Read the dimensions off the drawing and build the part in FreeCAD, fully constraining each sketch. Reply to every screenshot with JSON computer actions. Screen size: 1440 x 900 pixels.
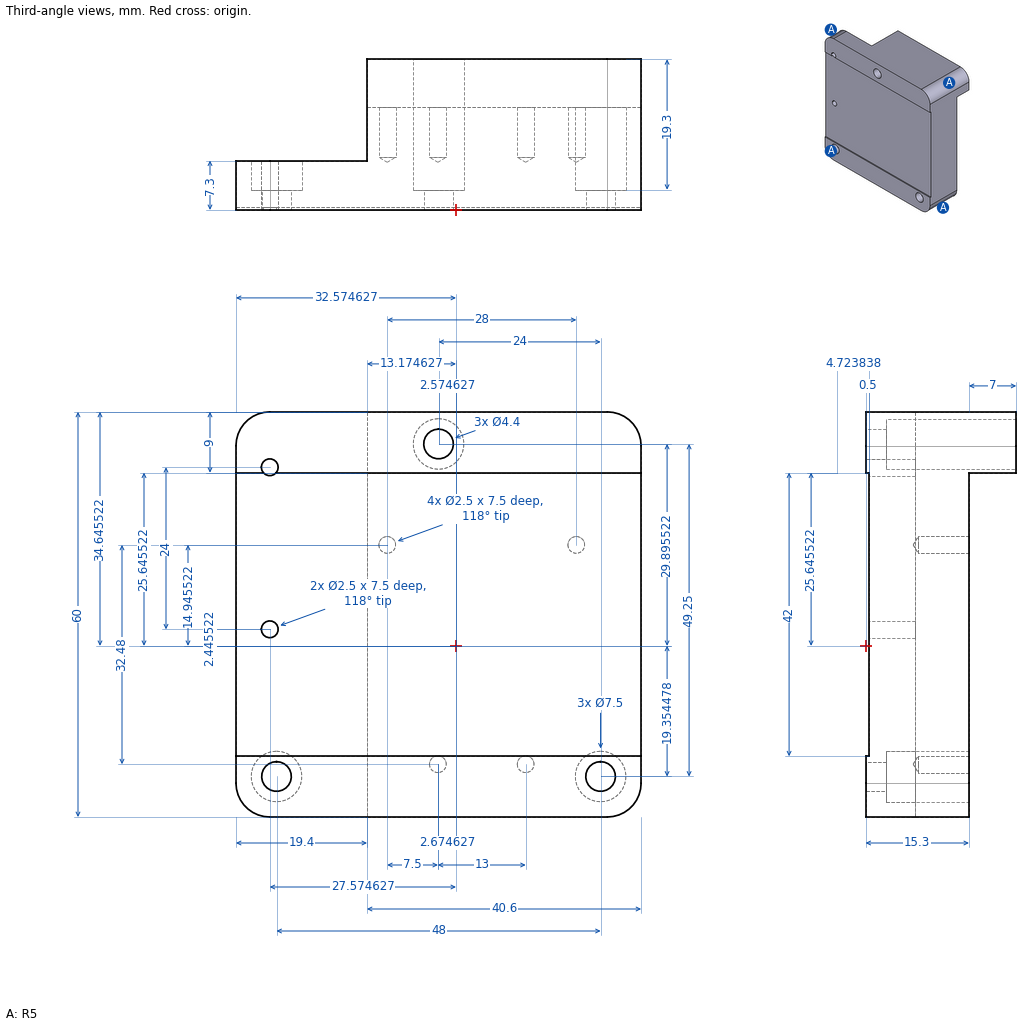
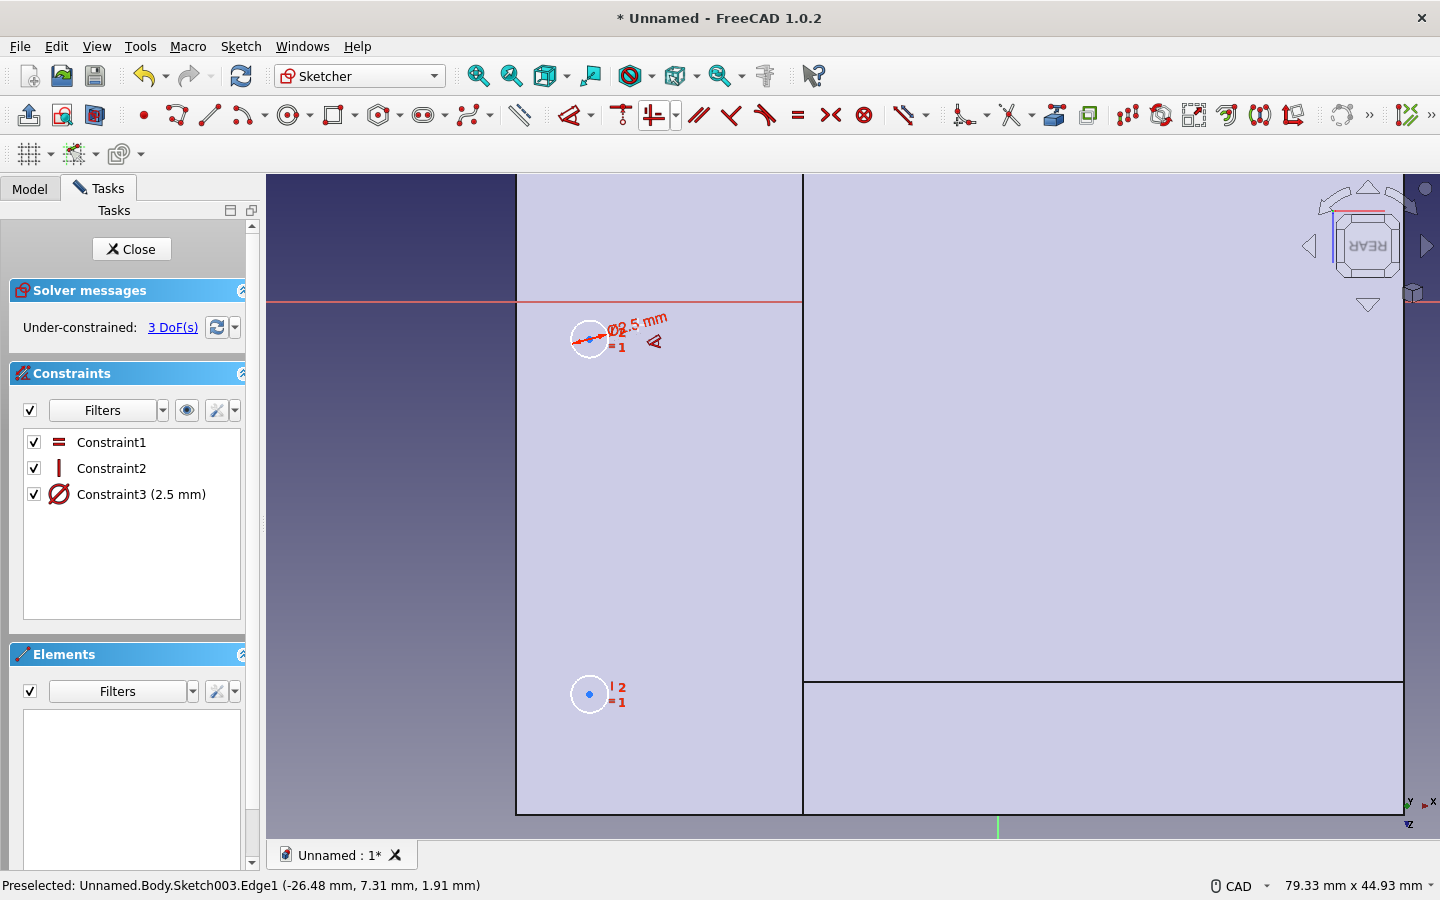
{"action": "left_click", "coordinate": [590, 339]}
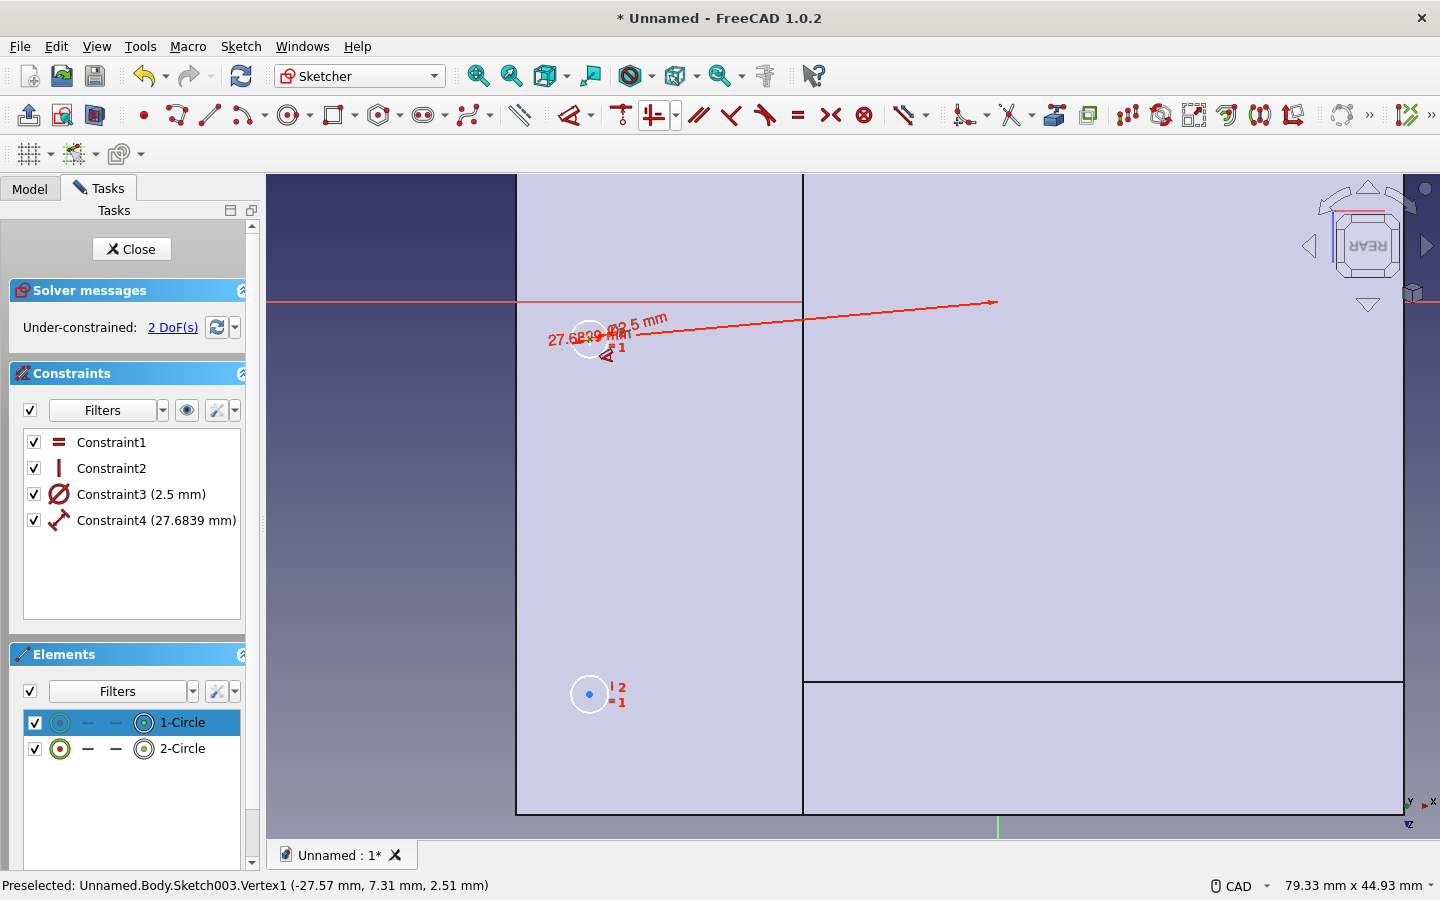
{"action": "left_click", "coordinate": [590, 694]}
{"action": "left_click", "coordinate": [556, 517]}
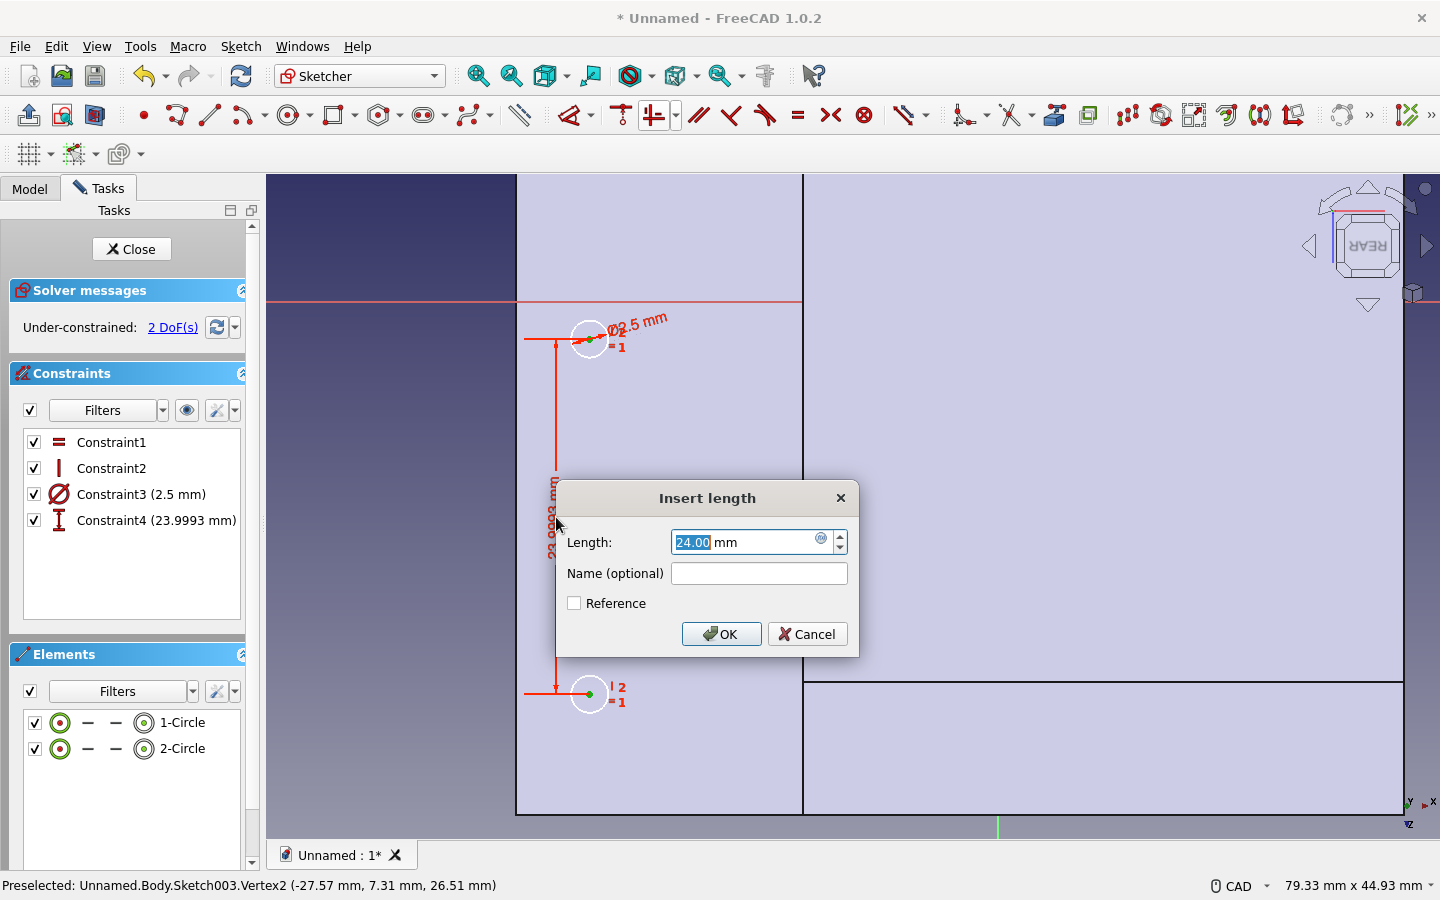
{"action": "type", "text": "24"}
{"action": "key", "text": "Return"}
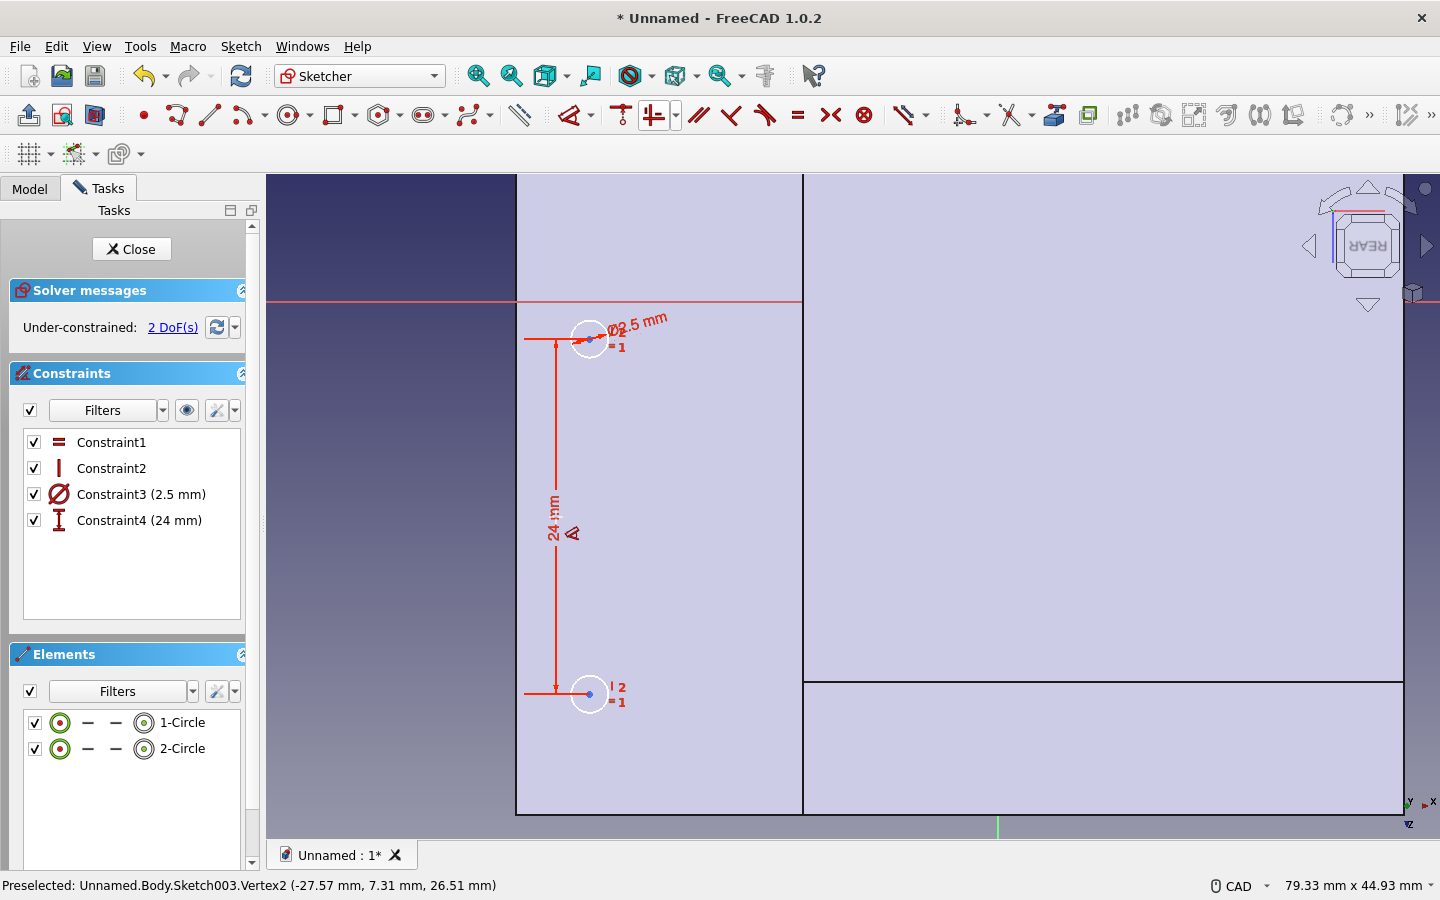
{"action": "left_click", "coordinate": [590, 339]}
{"action": "left_click", "coordinate": [1032, 321]}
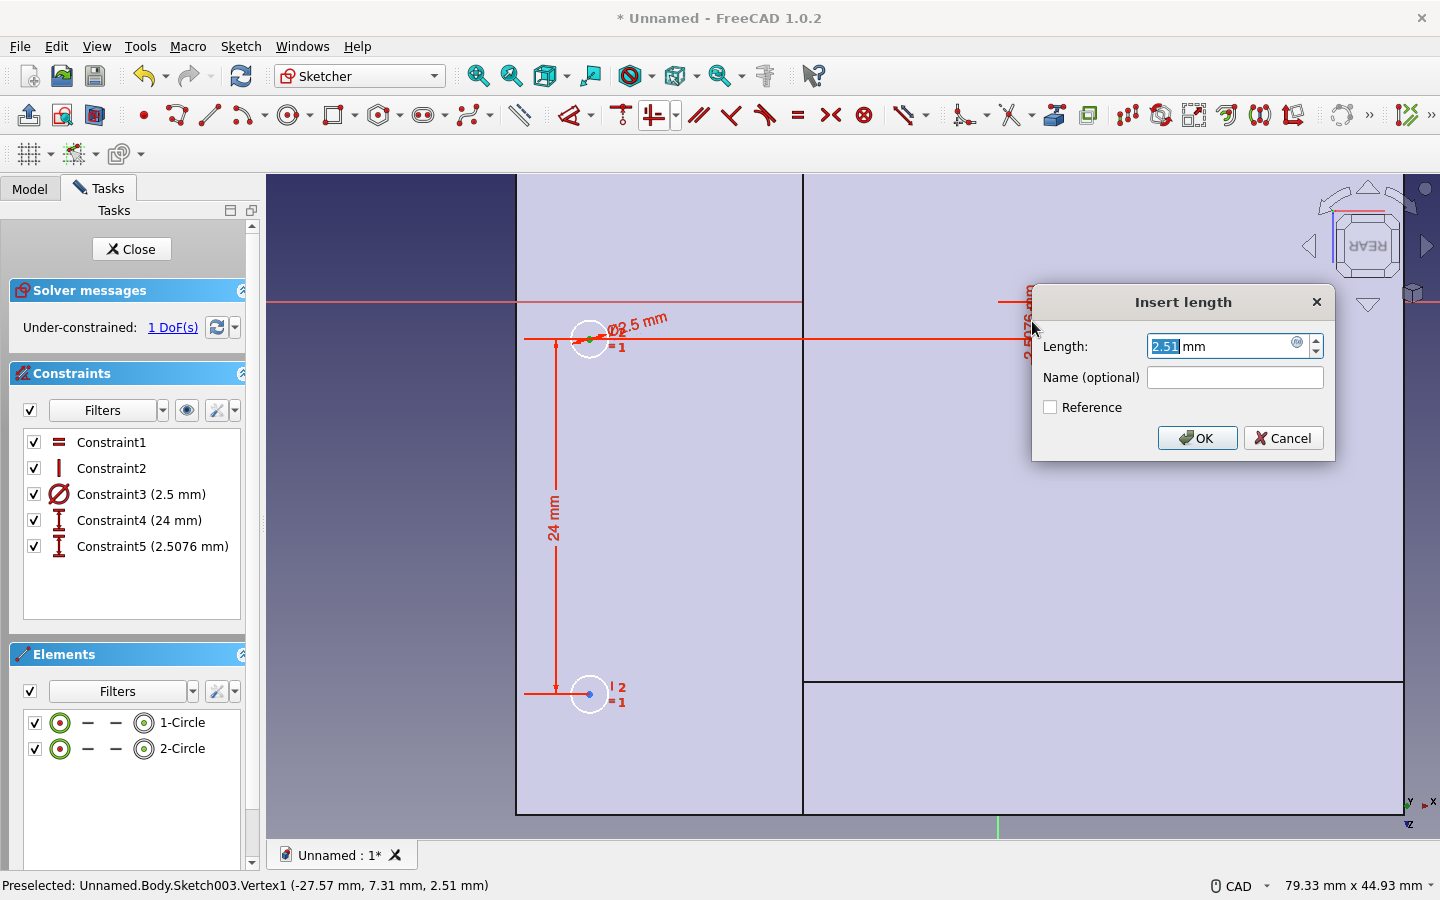
{"action": "type", "text": "2.445522"}
{"action": "key", "text": "Return"}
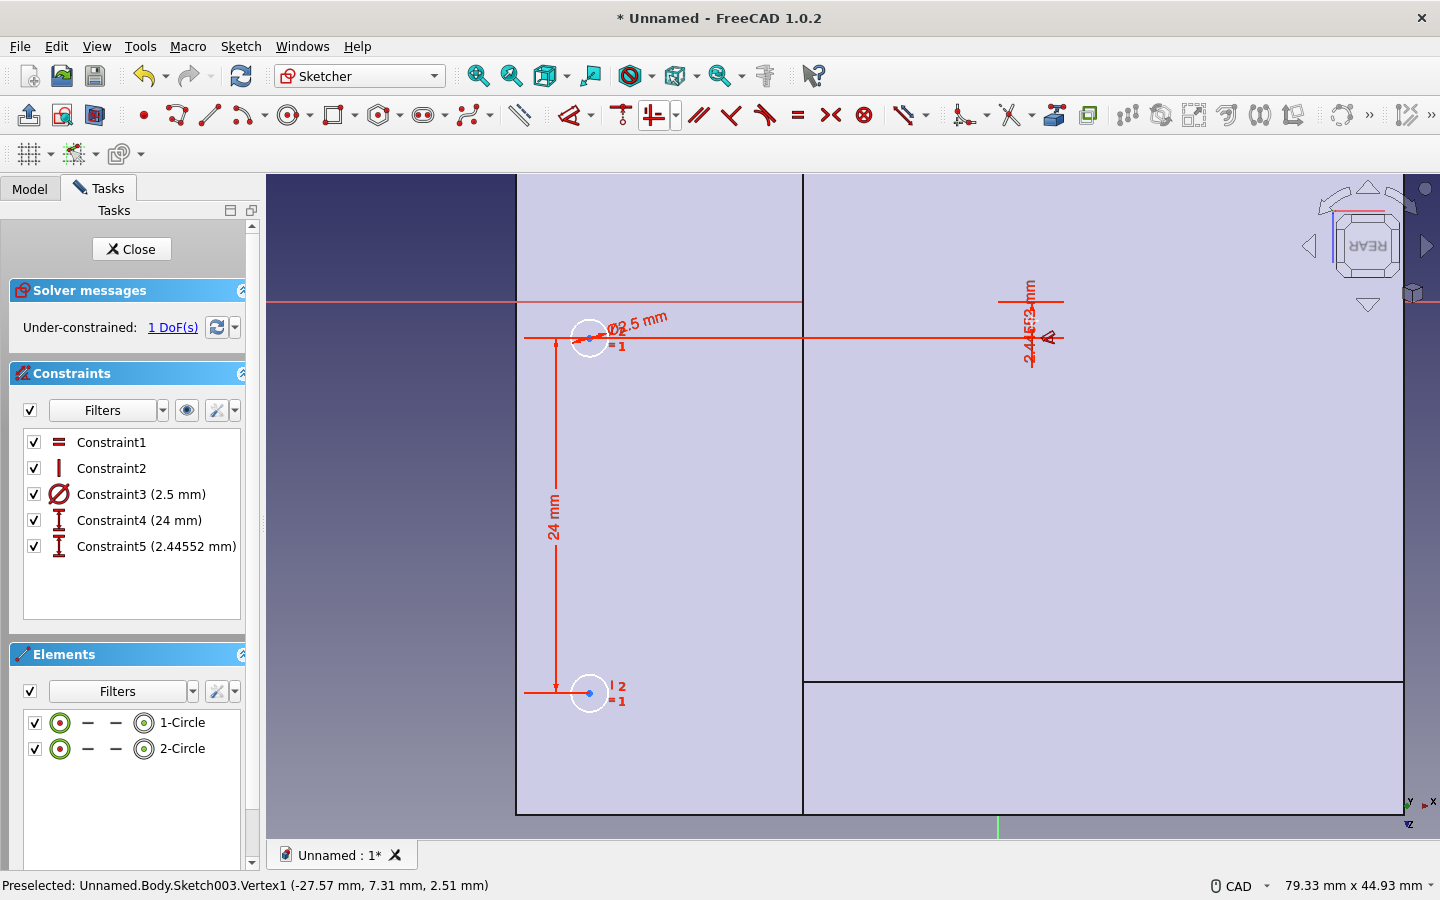
{"action": "left_click", "coordinate": [590, 338]}
{"action": "left_click", "coordinate": [794, 268]}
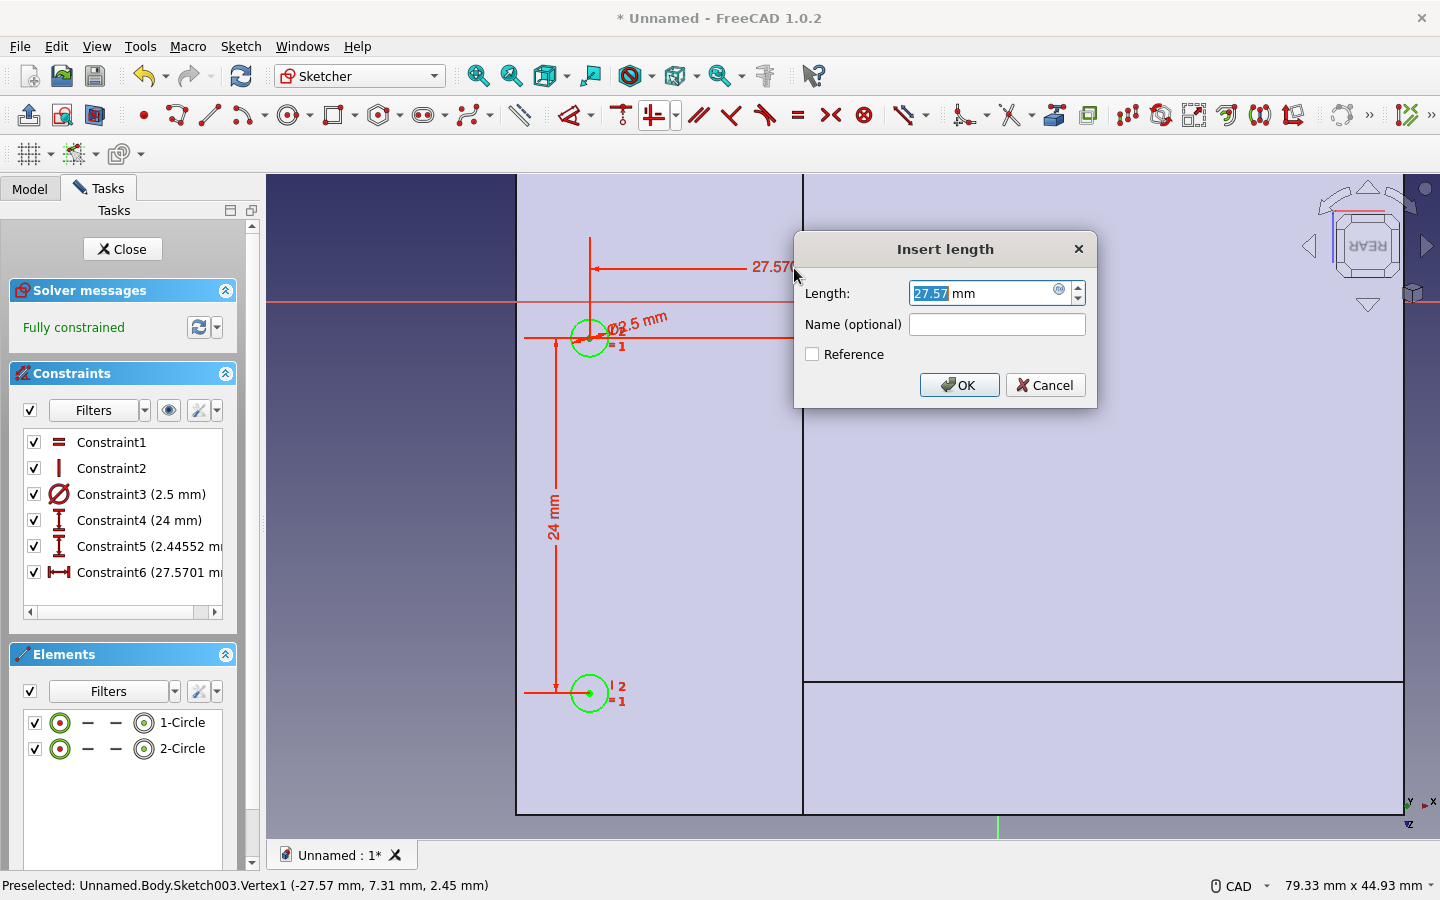
{"action": "type", "text": "27.574627"}
{"action": "key", "text": "Return"}
{"action": "key", "text": "Escape"}